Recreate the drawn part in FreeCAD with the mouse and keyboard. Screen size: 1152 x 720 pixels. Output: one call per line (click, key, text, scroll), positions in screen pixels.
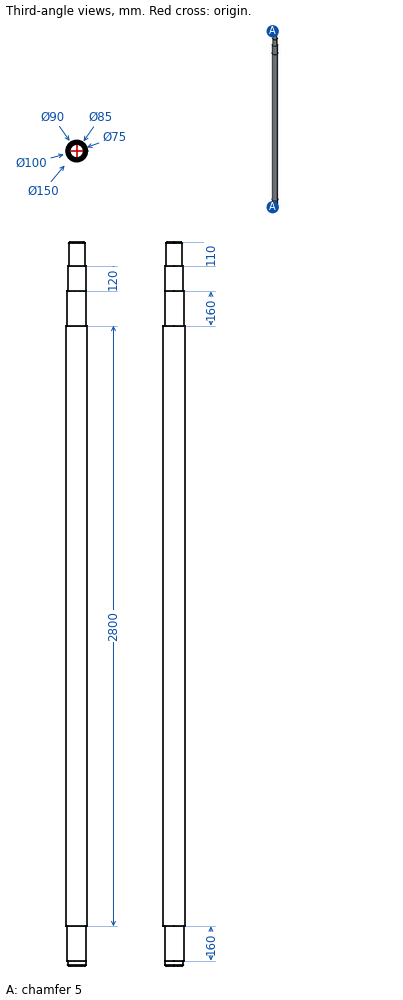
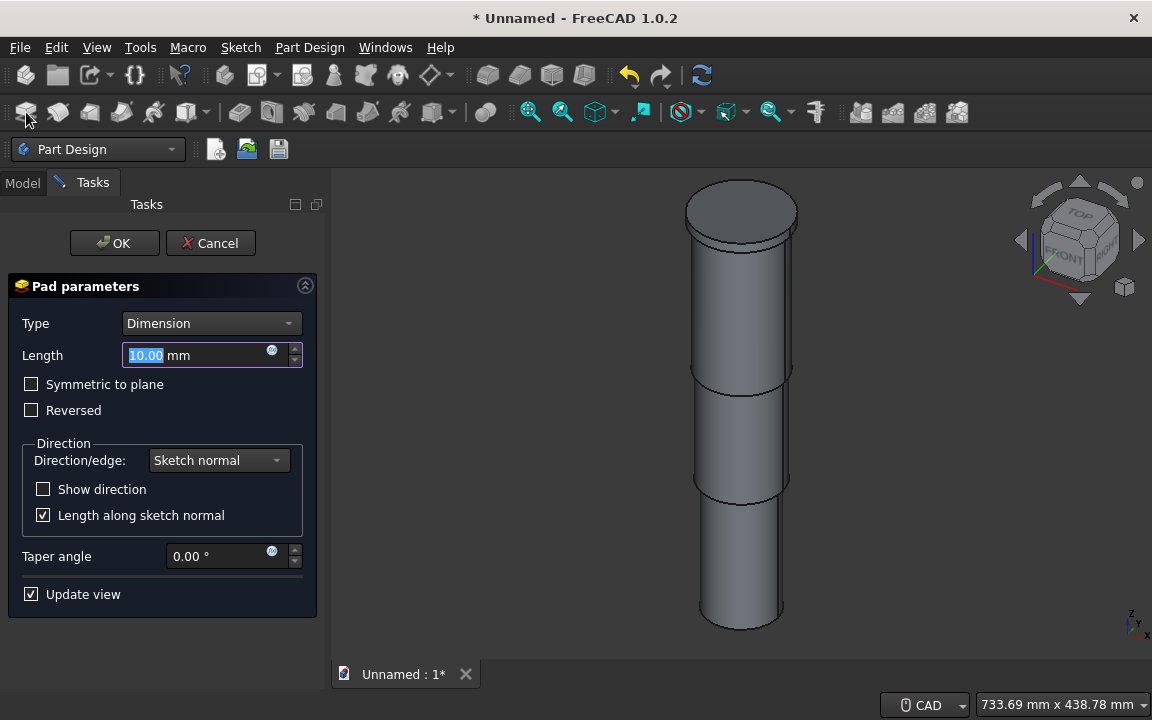
text(2800)
key(Tab)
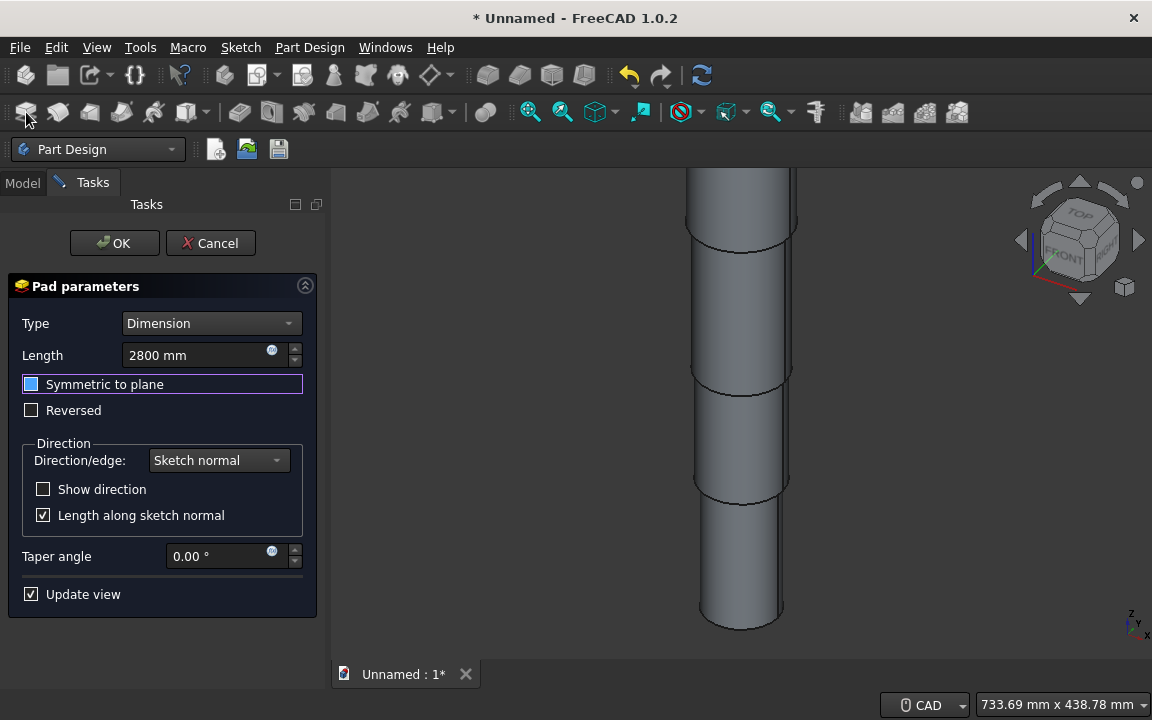
click(115, 243)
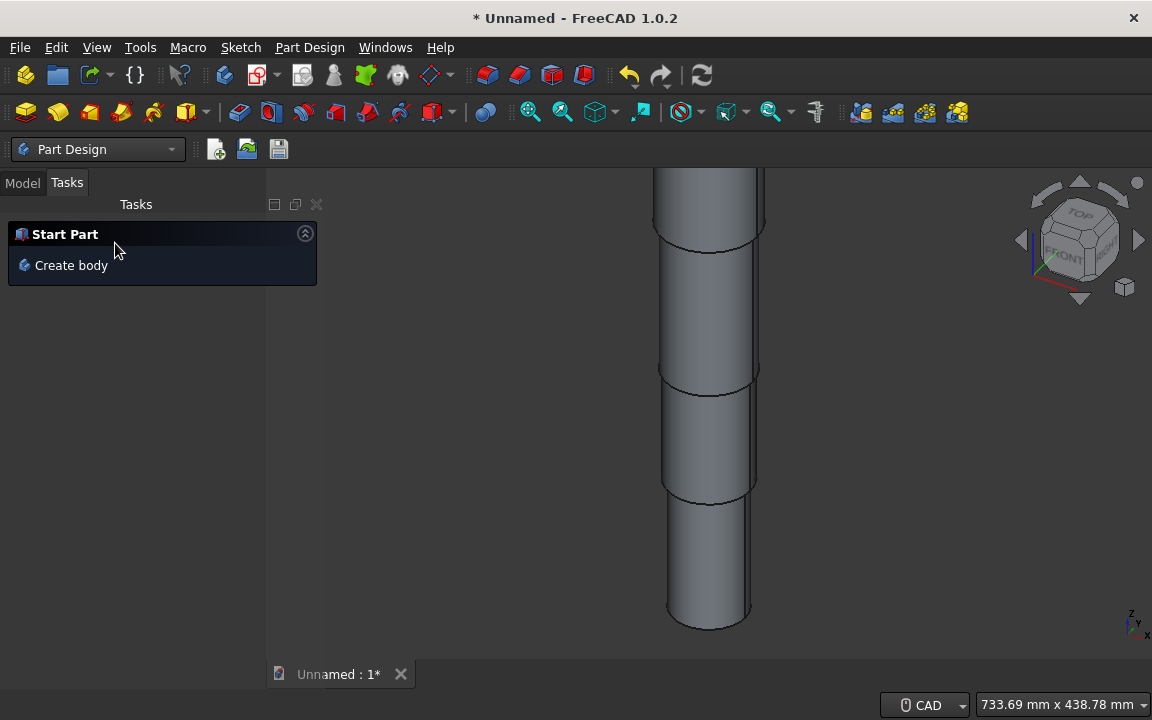
click(532, 112)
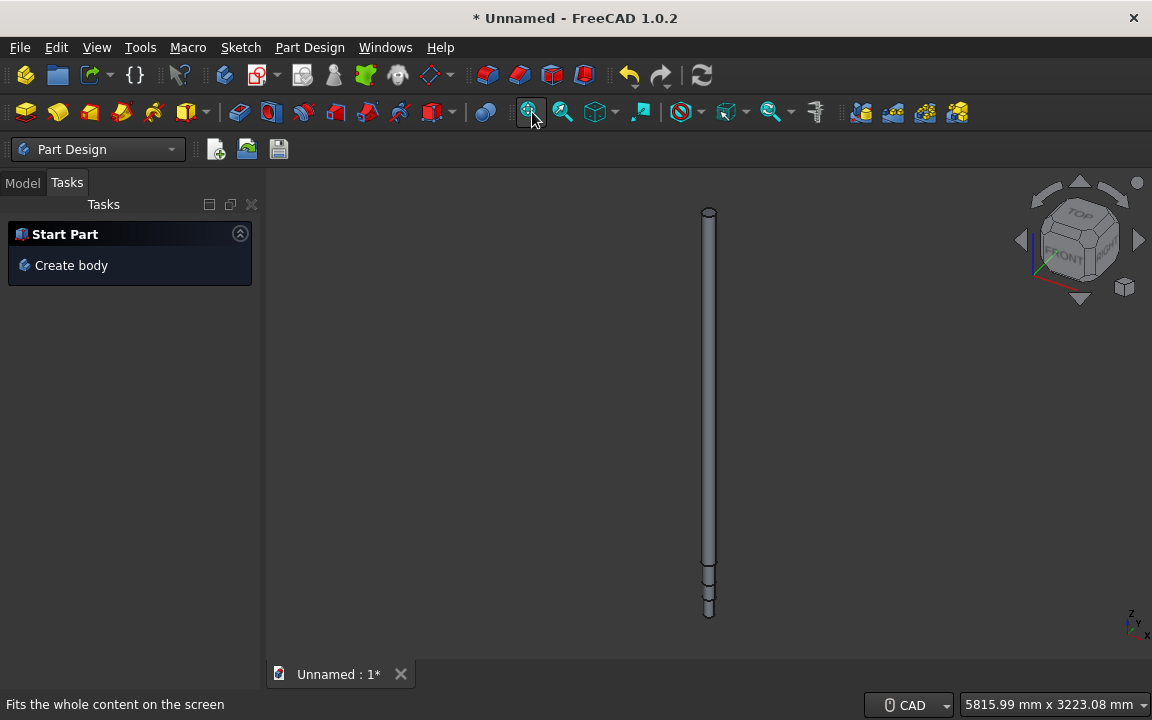
key(0)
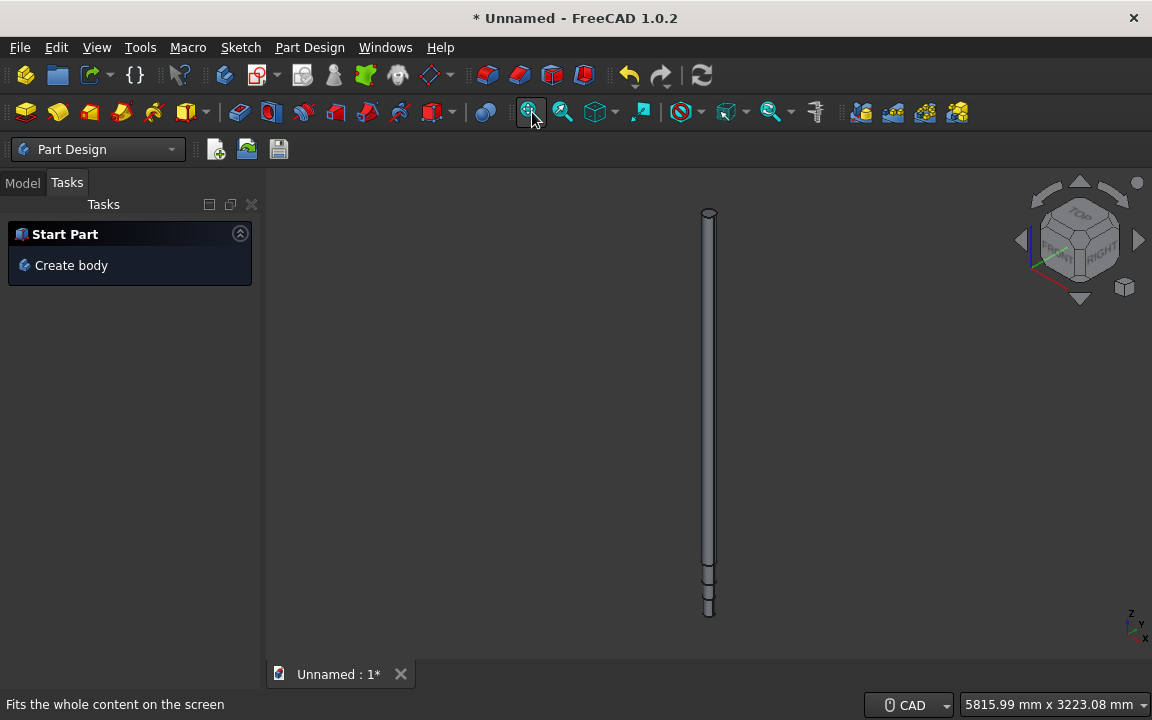
key(2)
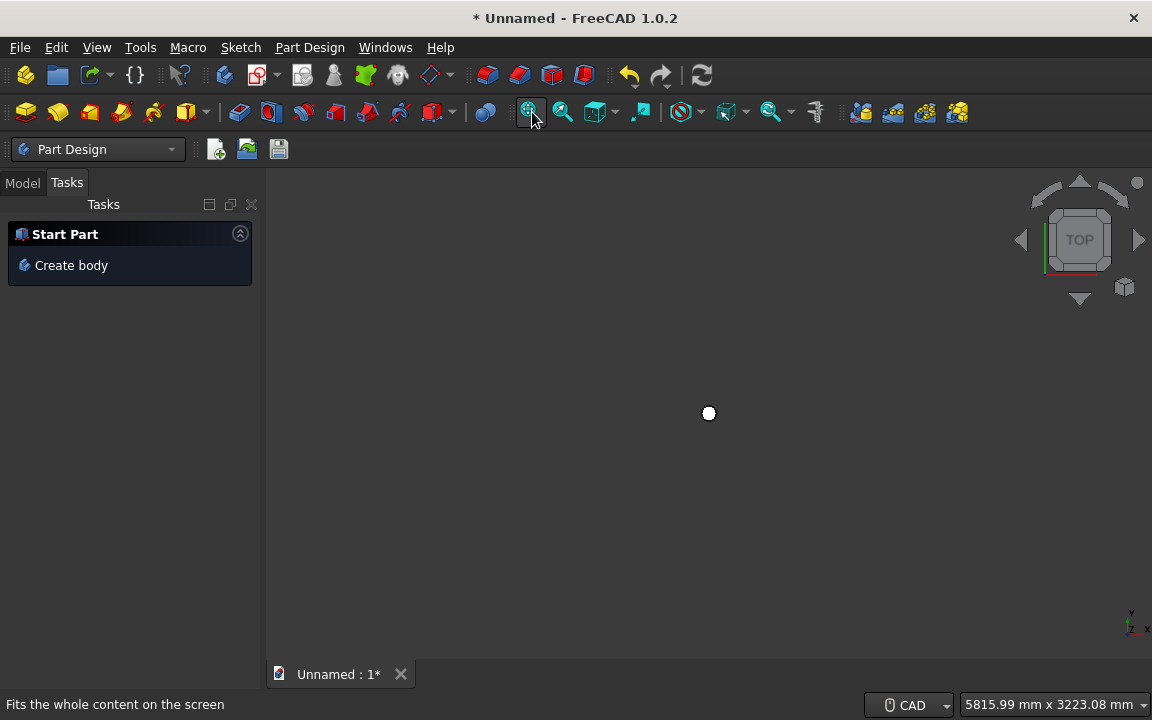
click(532, 112)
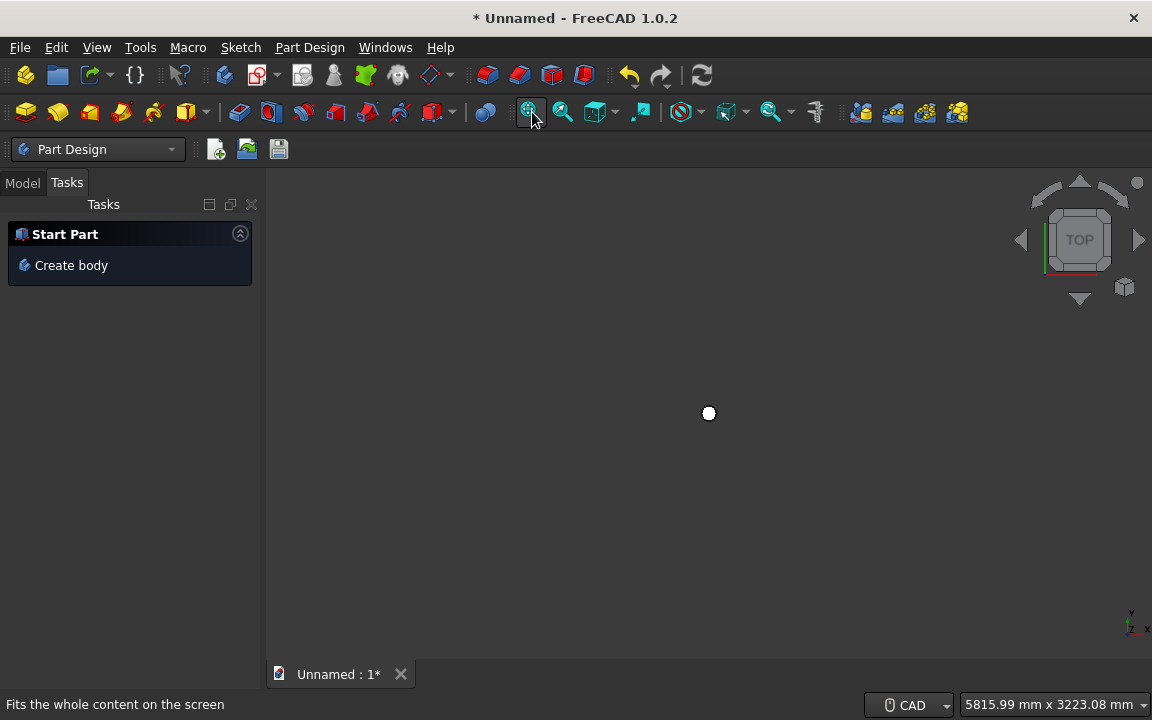
key(1)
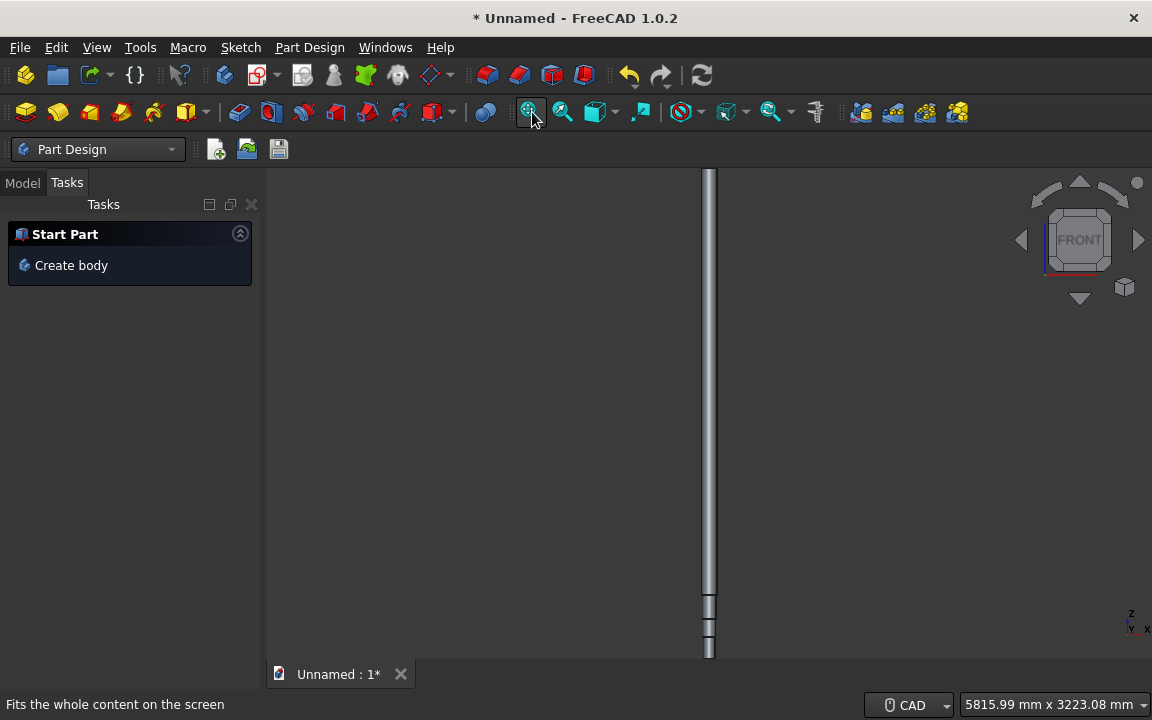
click(532, 112)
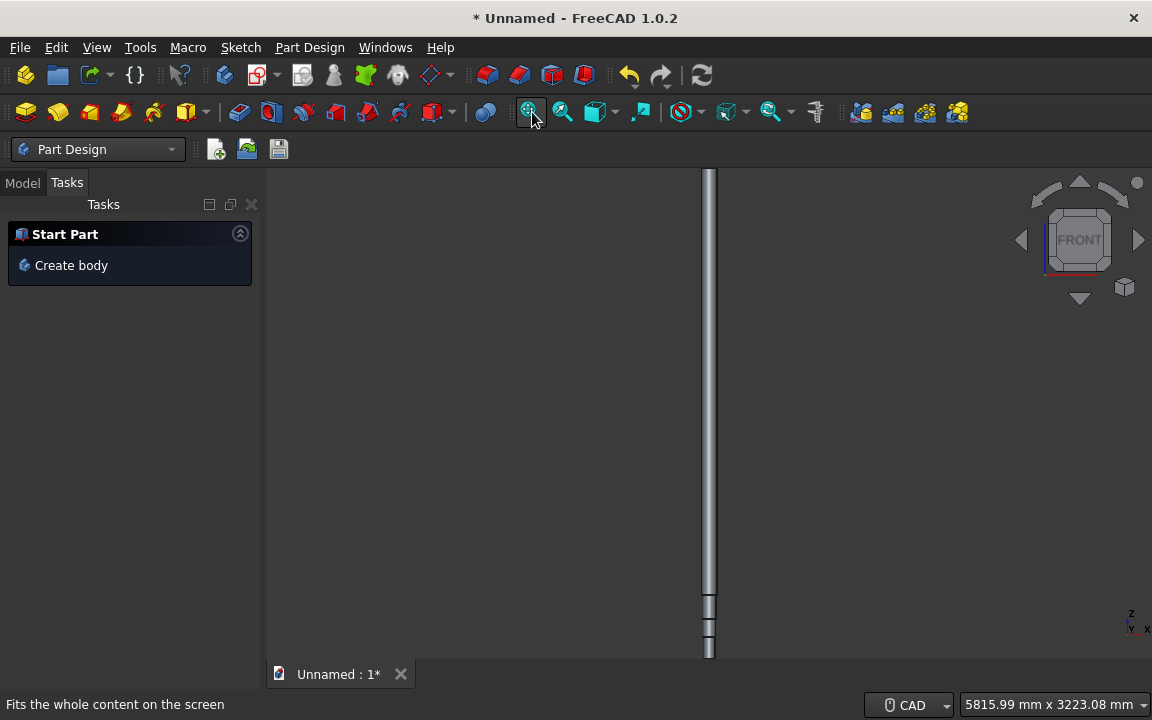
click(23, 182)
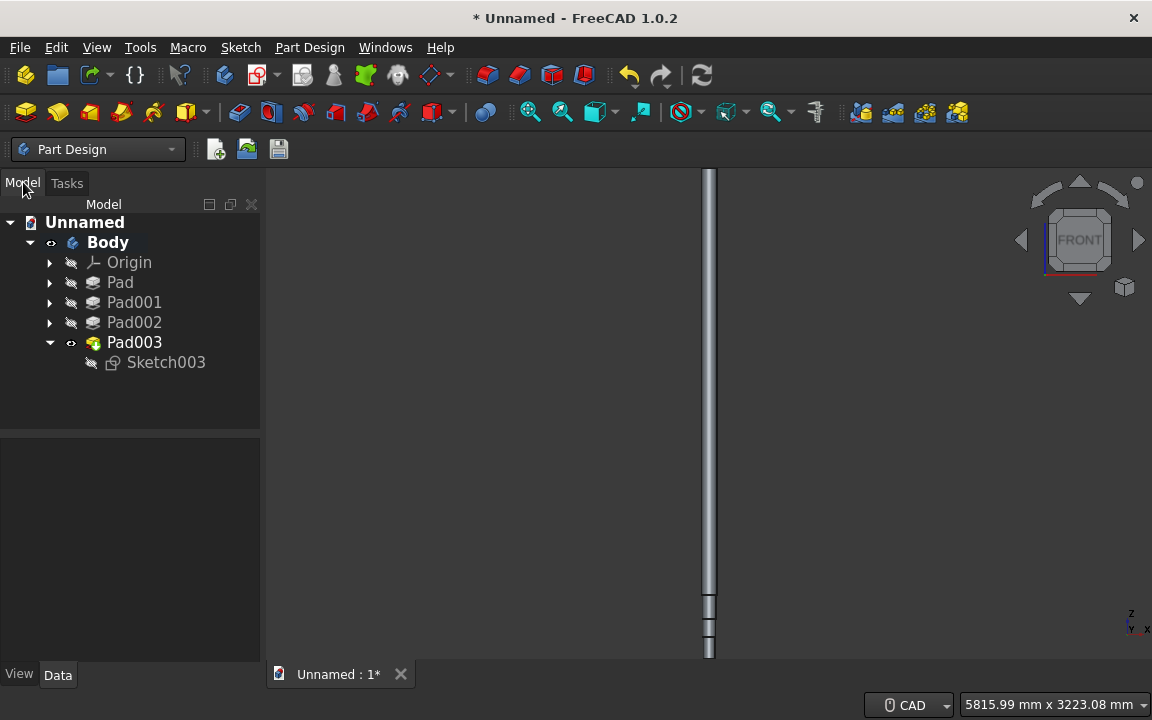
click(50, 263)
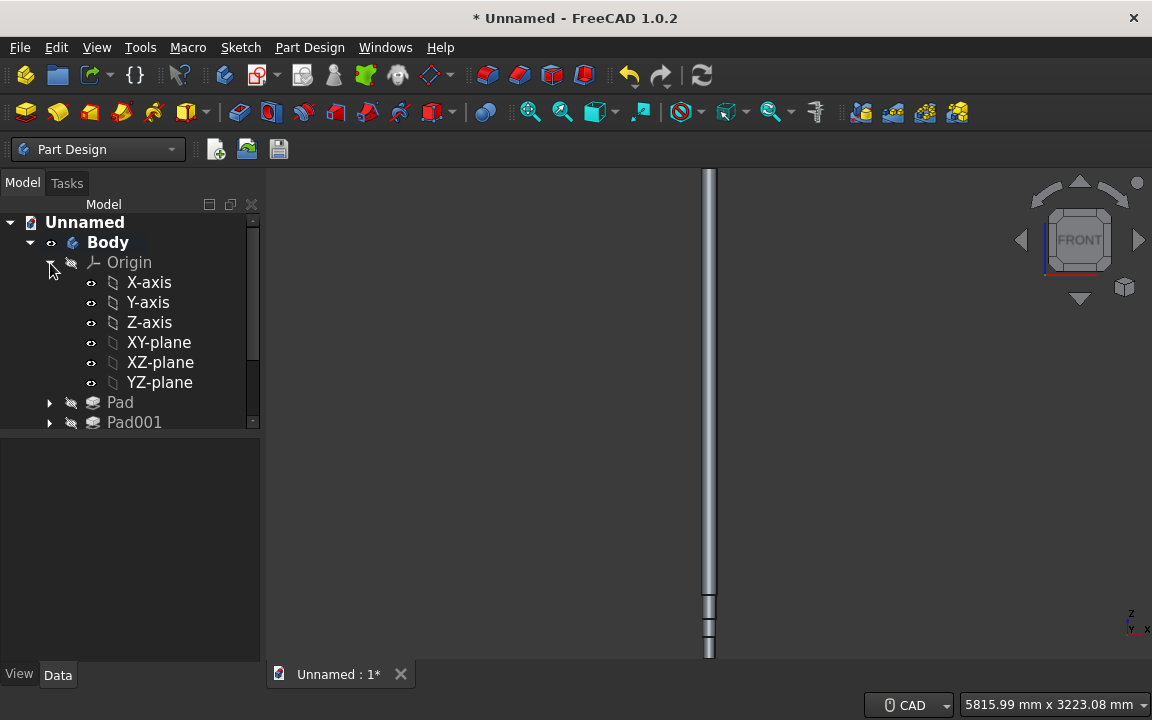
click(136, 343)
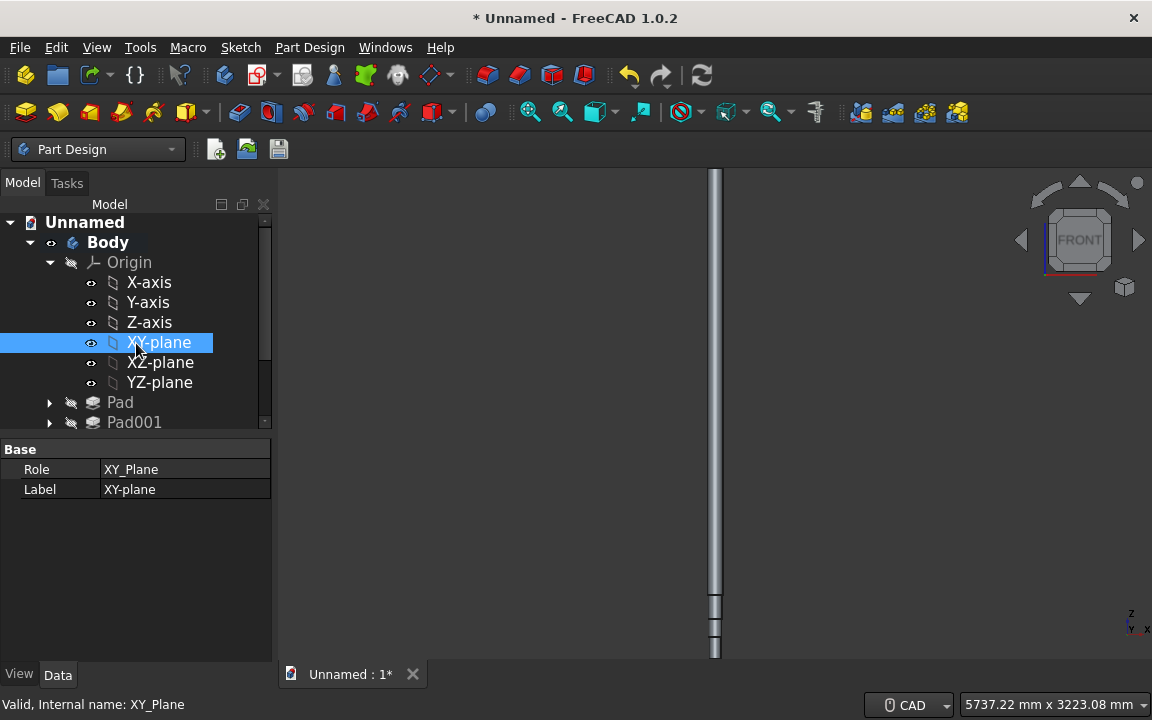
click(430, 76)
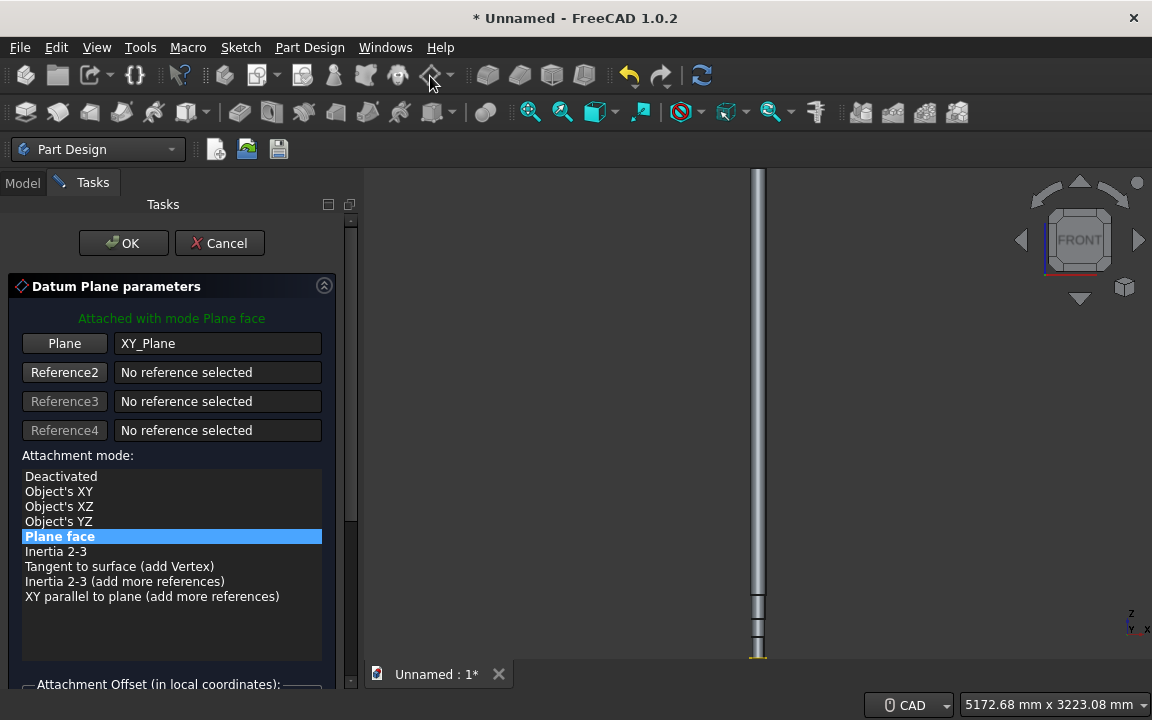
scroll(351, 451, down, 3)